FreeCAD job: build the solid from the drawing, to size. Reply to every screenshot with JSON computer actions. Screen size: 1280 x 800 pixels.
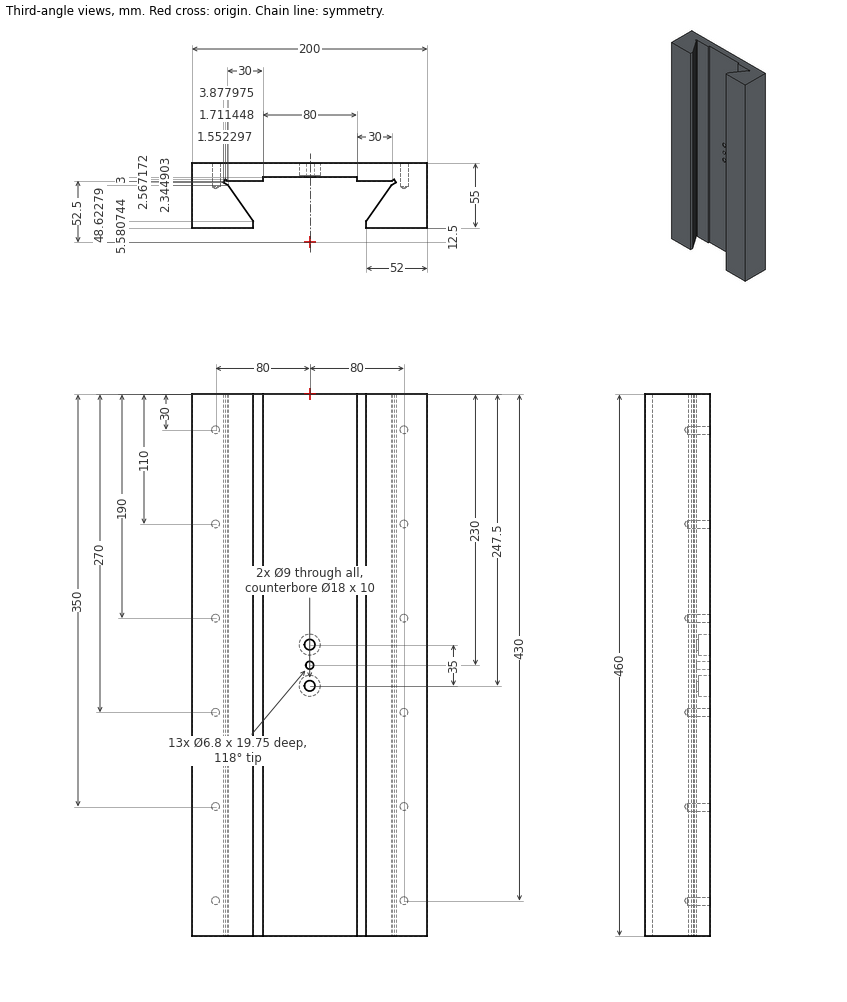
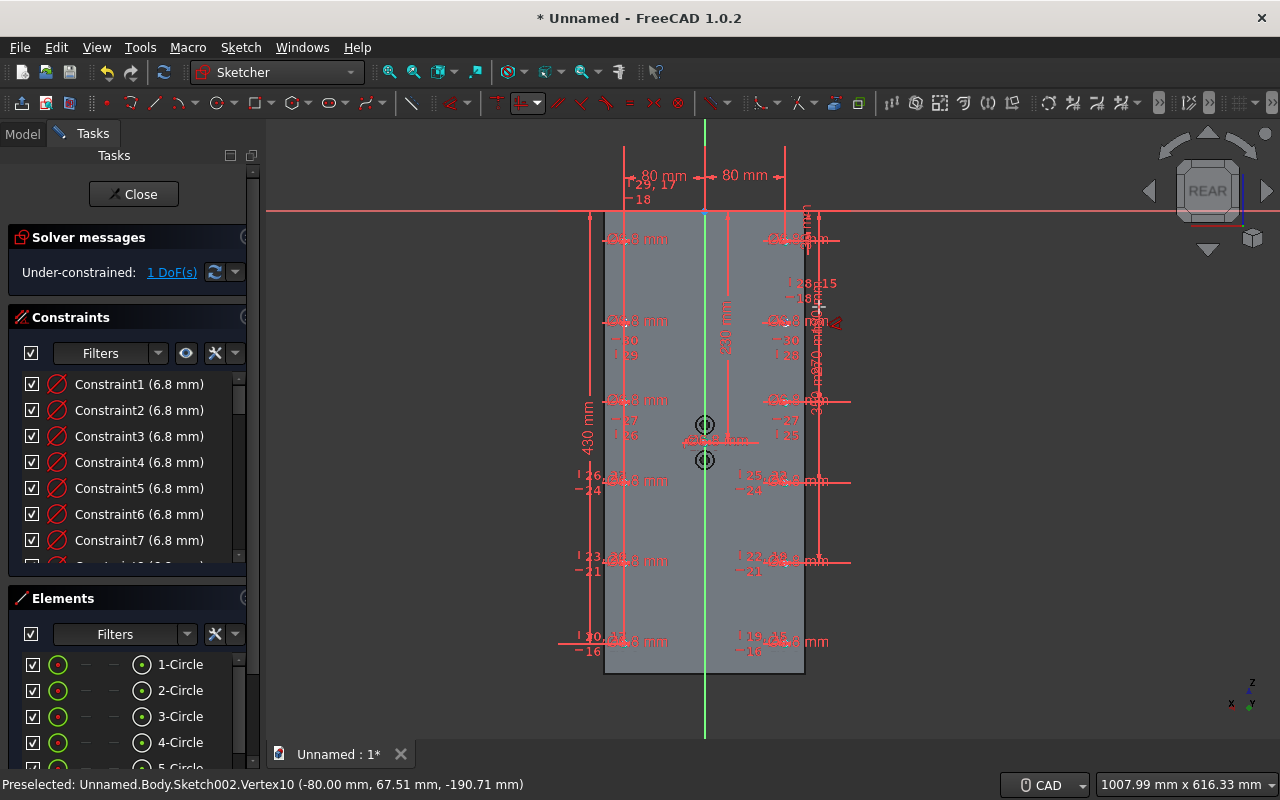
{"action": "left_click", "coordinate": [785, 323]}
{"action": "left_click", "coordinate": [819, 267]}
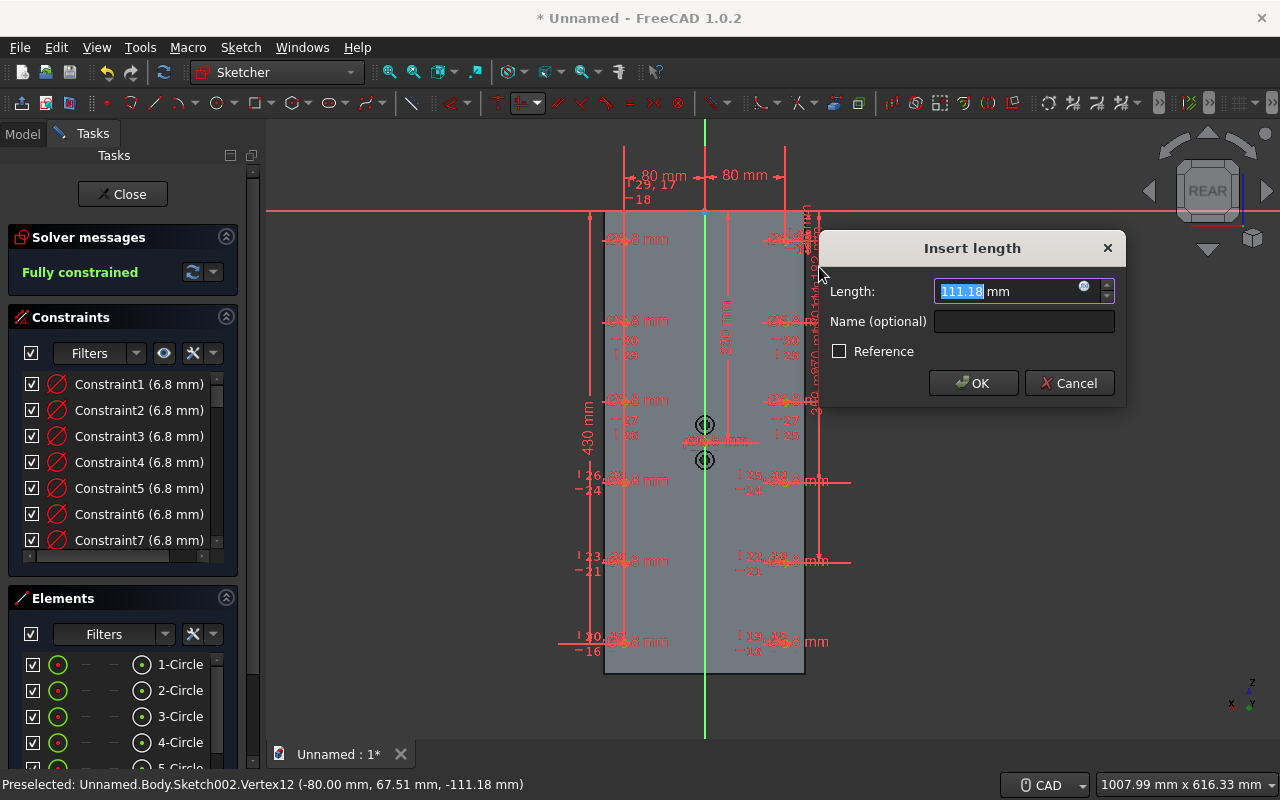
{"action": "type", "text": "110"}
{"action": "key", "text": "Return"}
{"action": "key", "text": "Escape"}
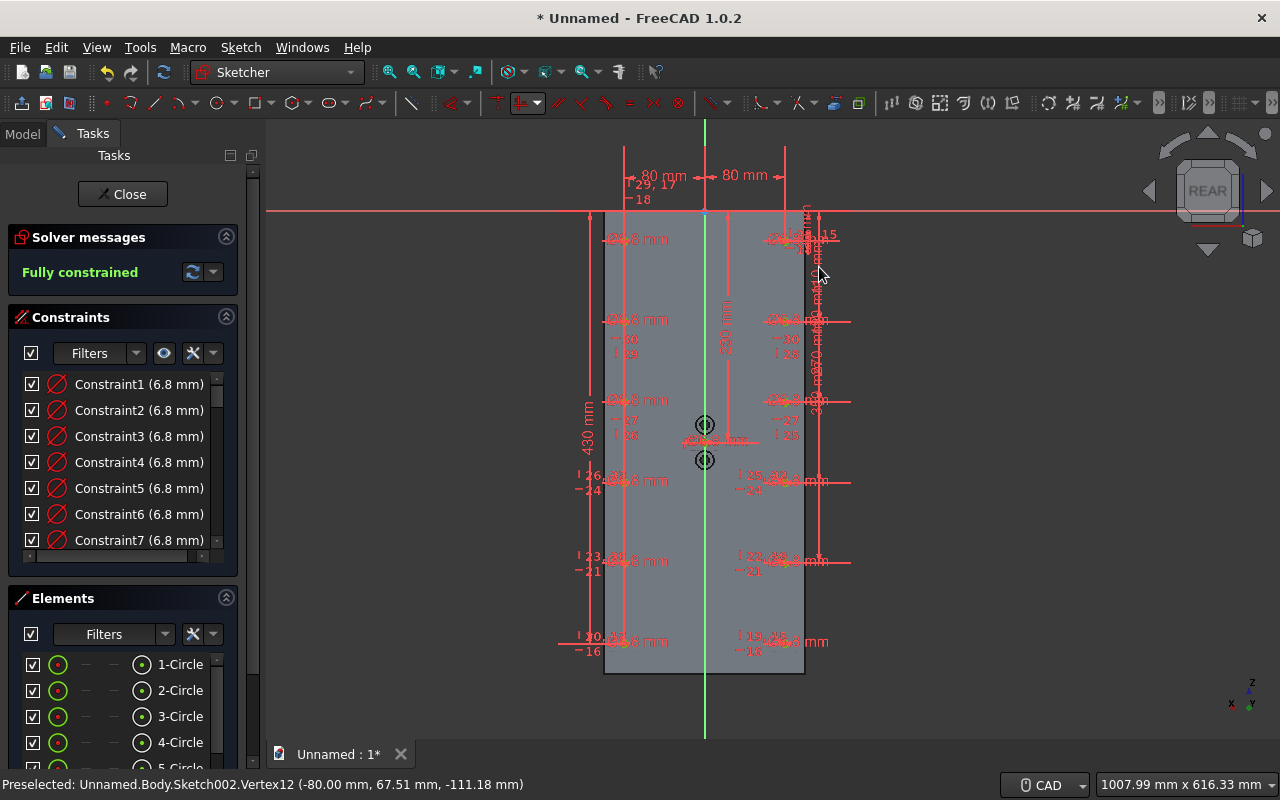
{"action": "left_click", "coordinate": [123, 194]}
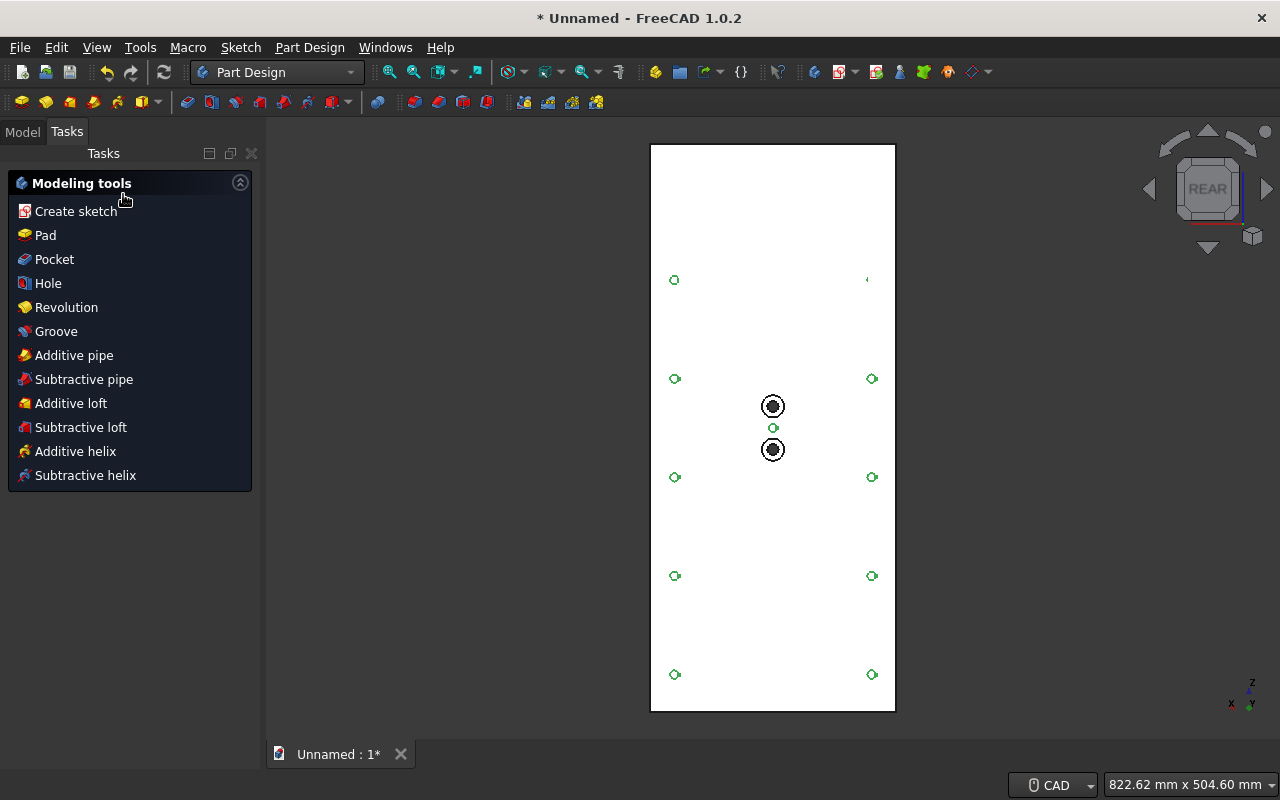
{"action": "left_click", "coordinate": [212, 102]}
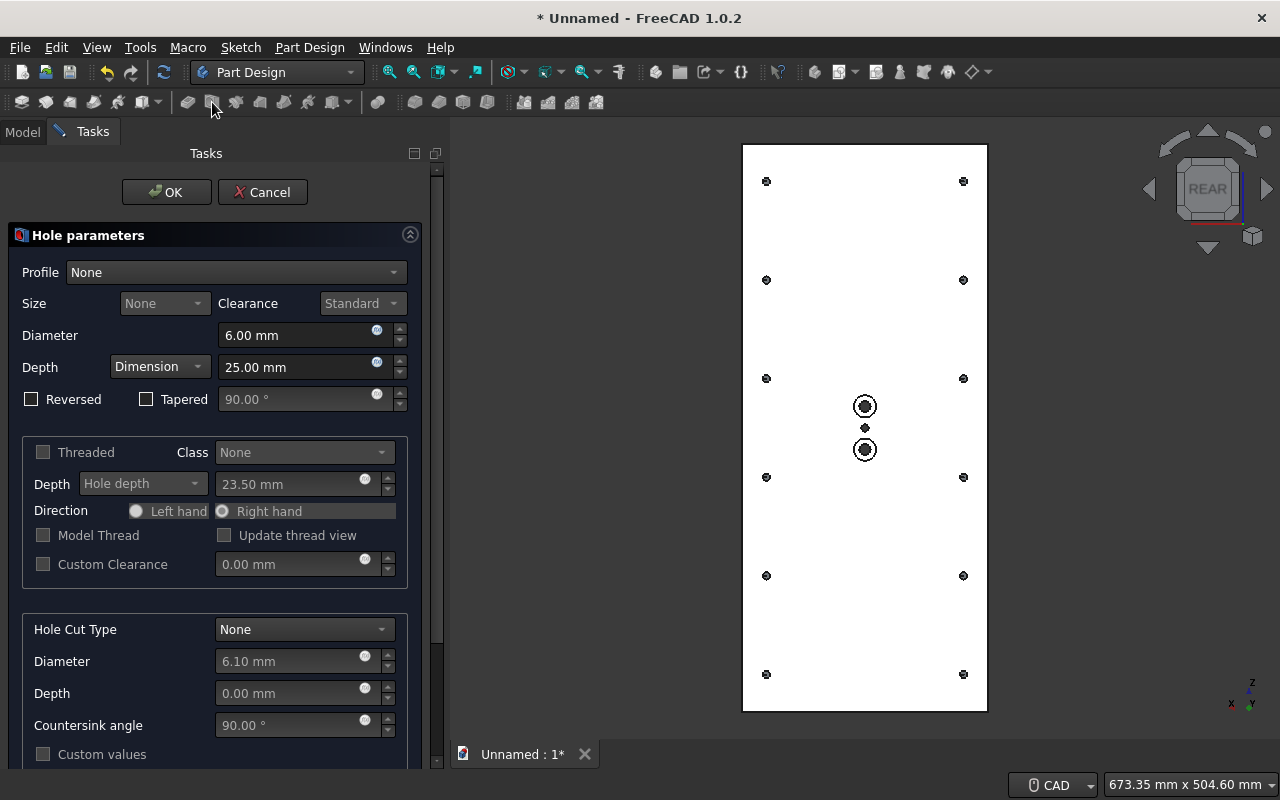
{"action": "triple_click", "coordinate": [305, 335]}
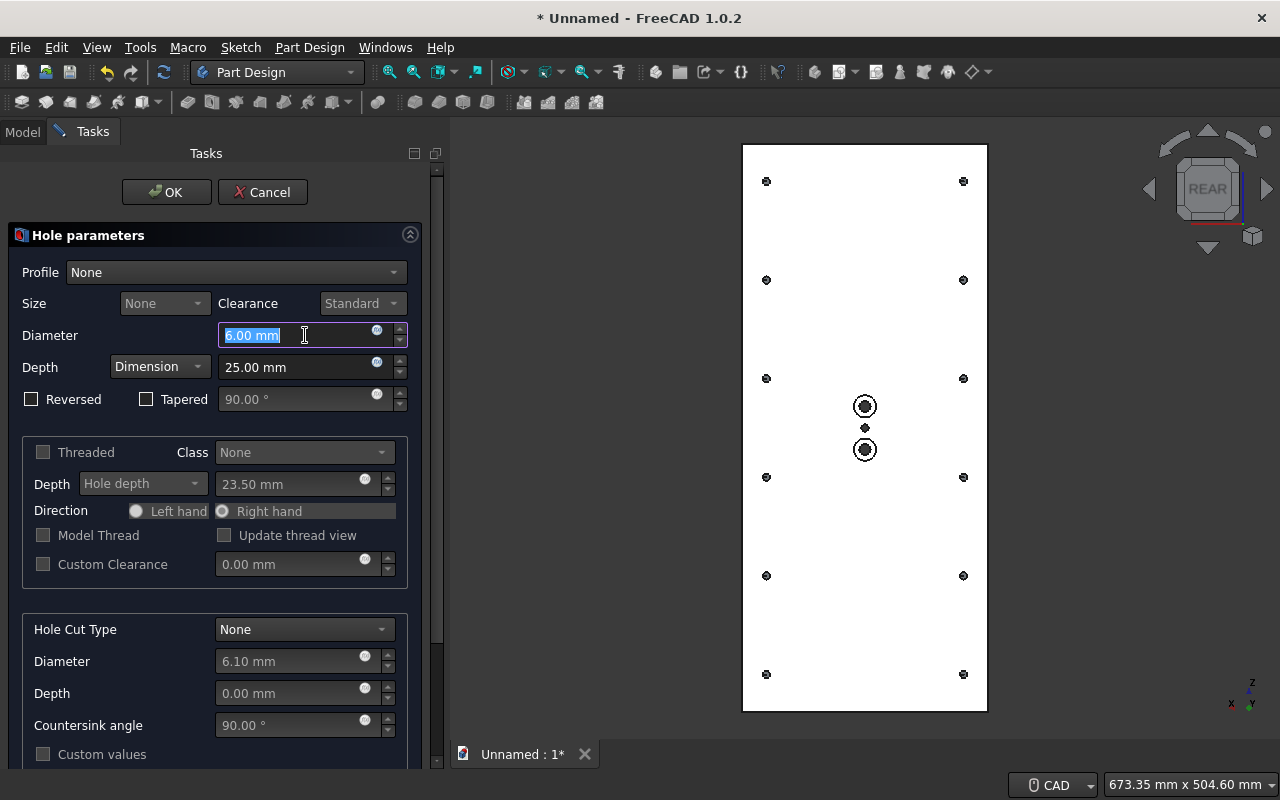
{"action": "type", "text": "6.8"}
{"action": "key", "text": "Tab"}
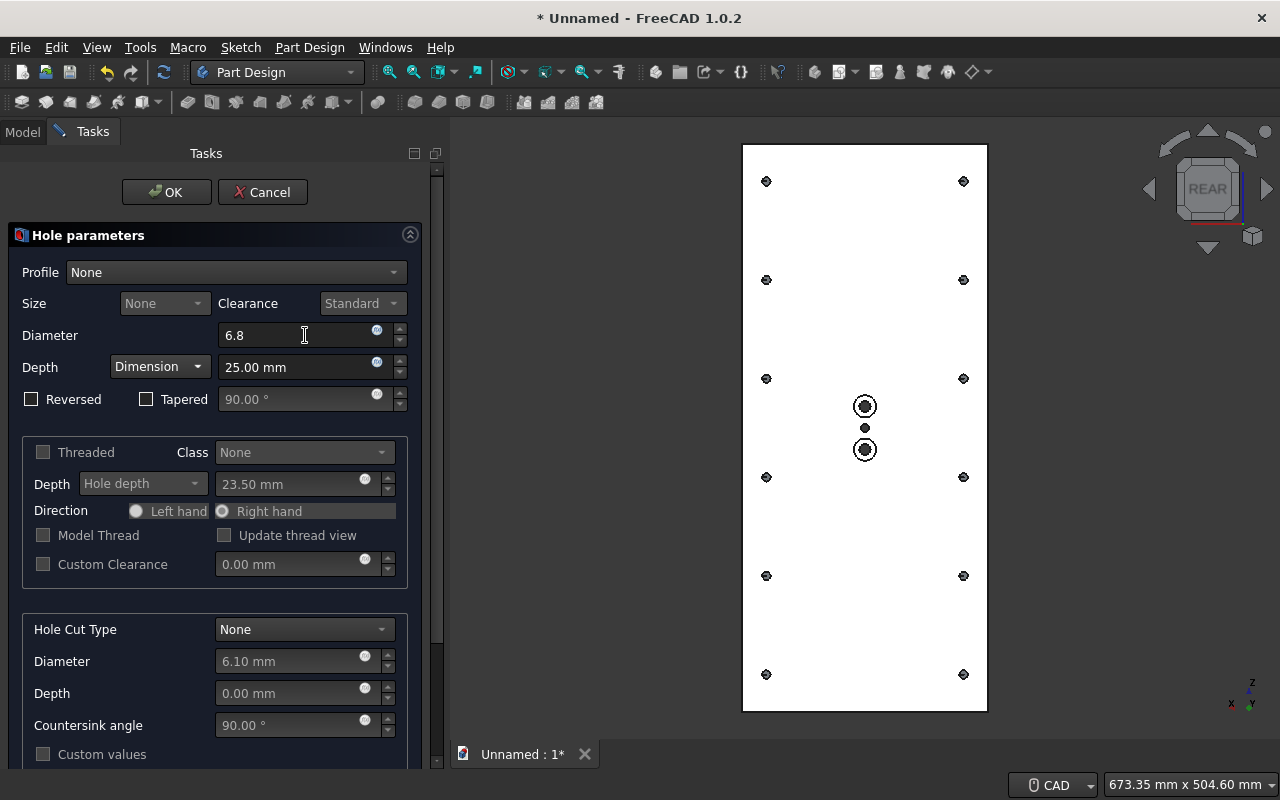
{"action": "triple_click", "coordinate": [305, 367]}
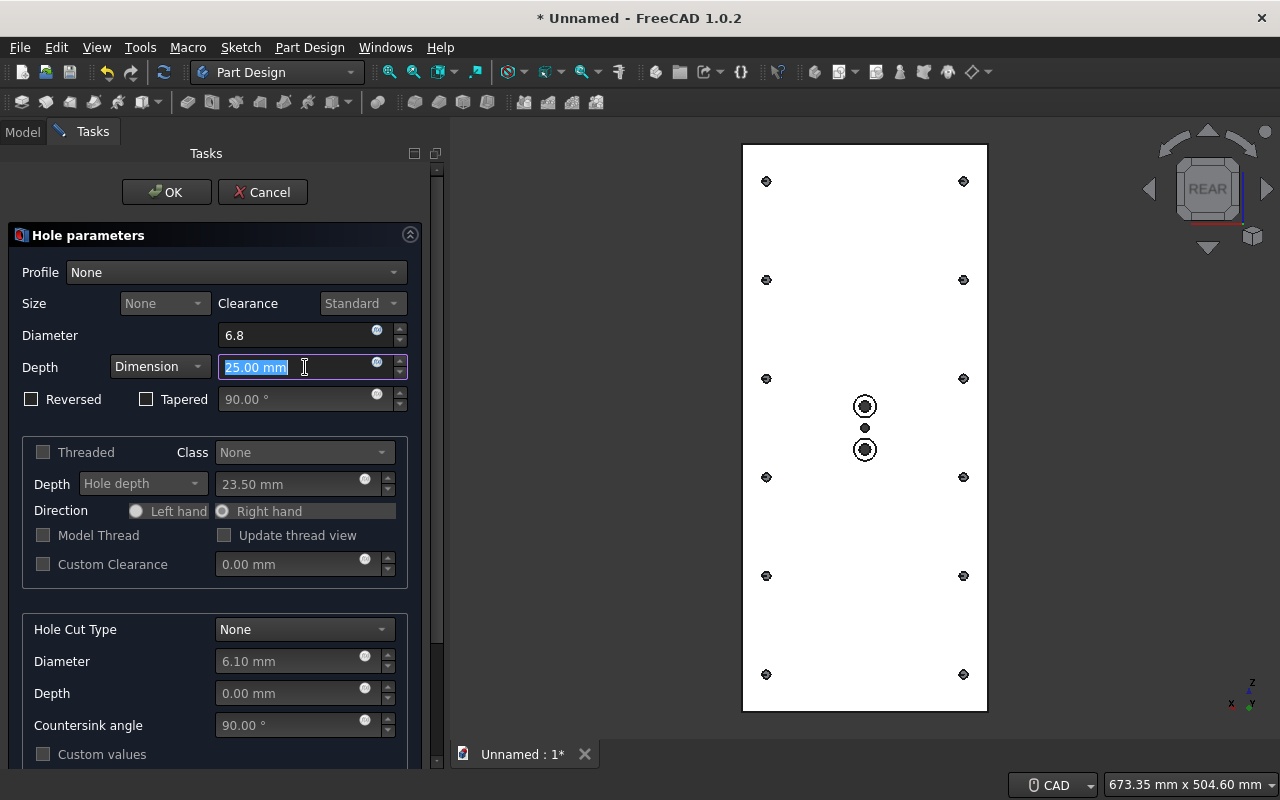
{"action": "type", "text": "19.75"}
{"action": "key", "text": "Tab"}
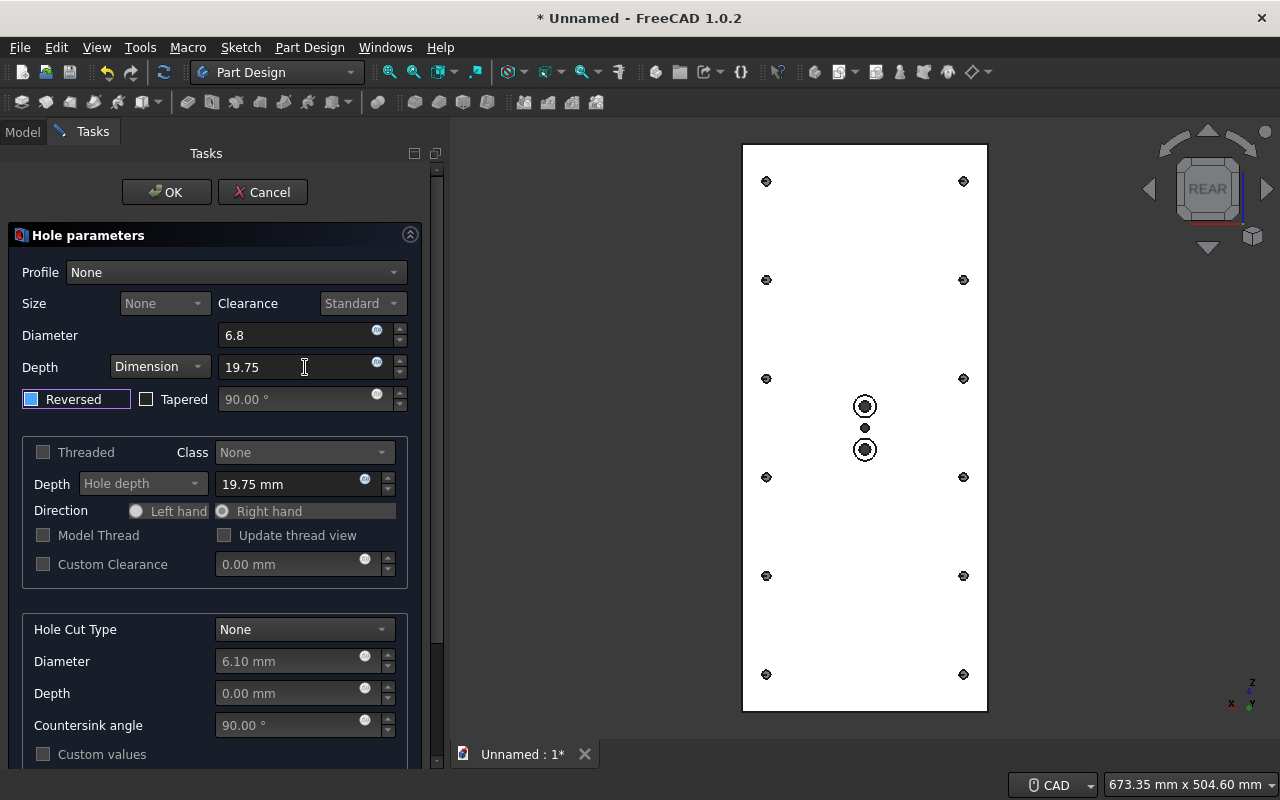
{"action": "left_click", "coordinate": [167, 192]}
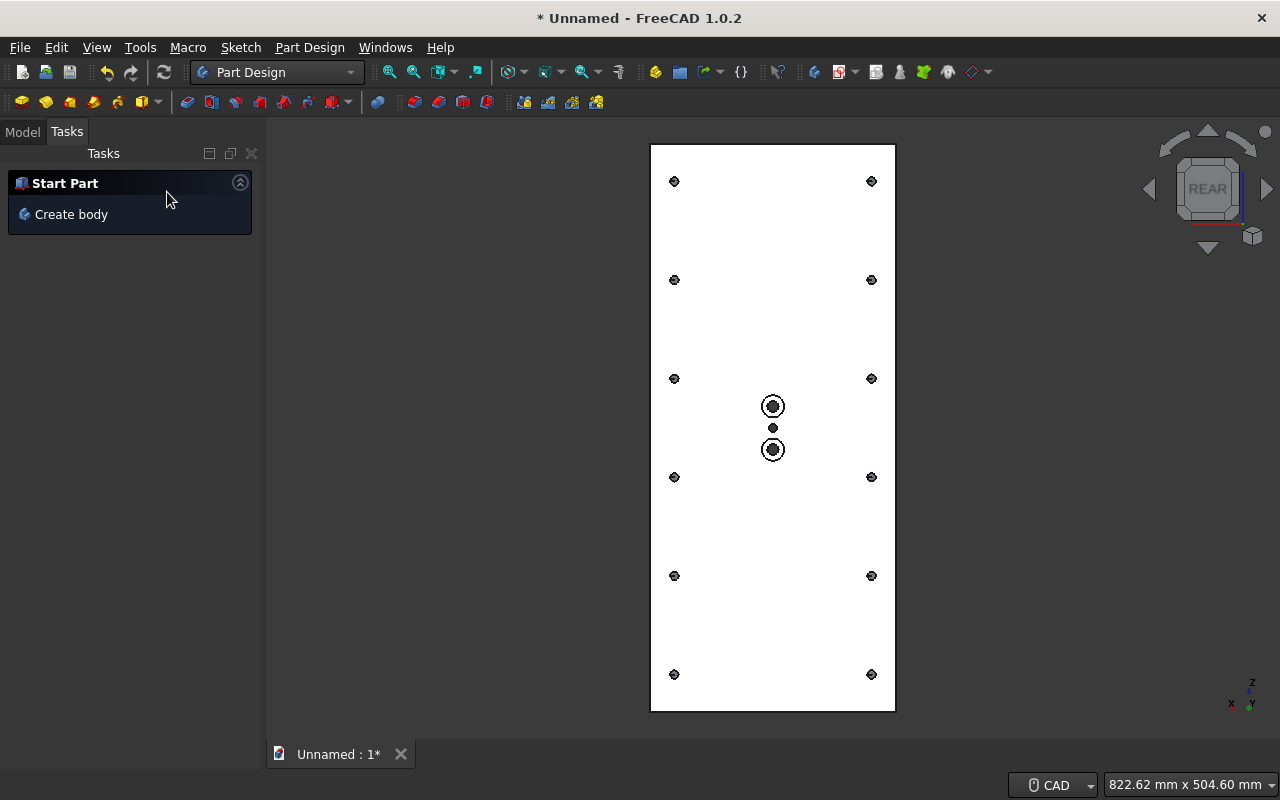
{"action": "key", "text": "0"}